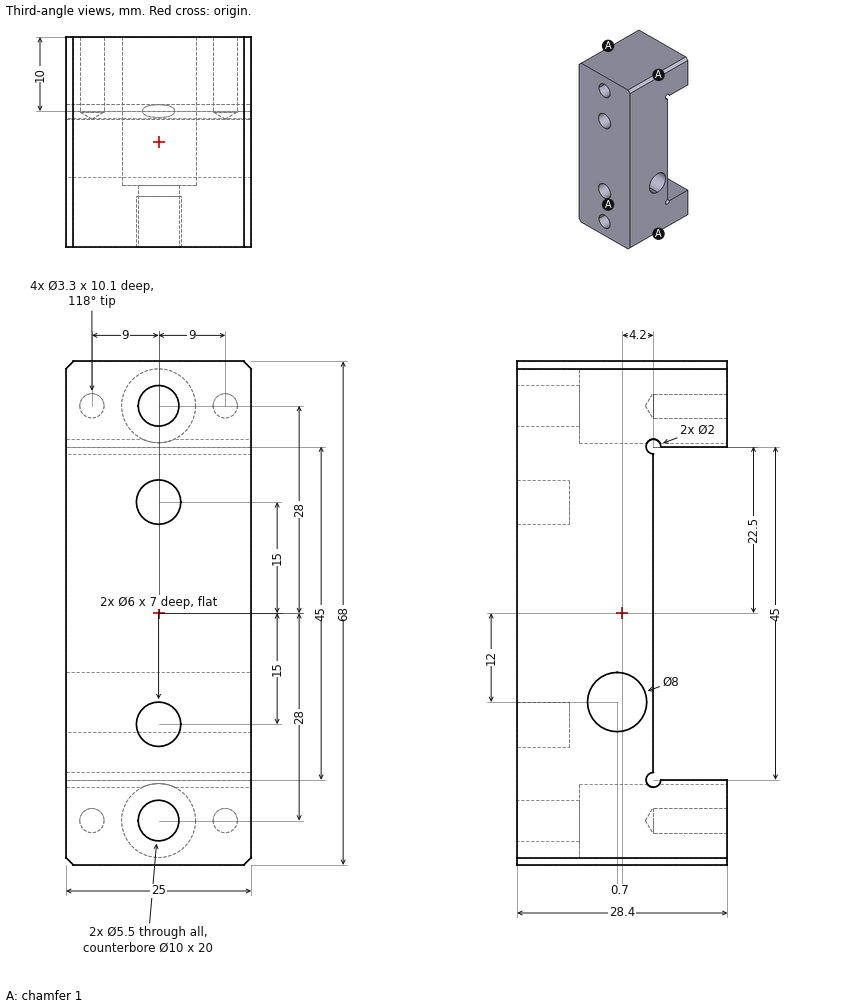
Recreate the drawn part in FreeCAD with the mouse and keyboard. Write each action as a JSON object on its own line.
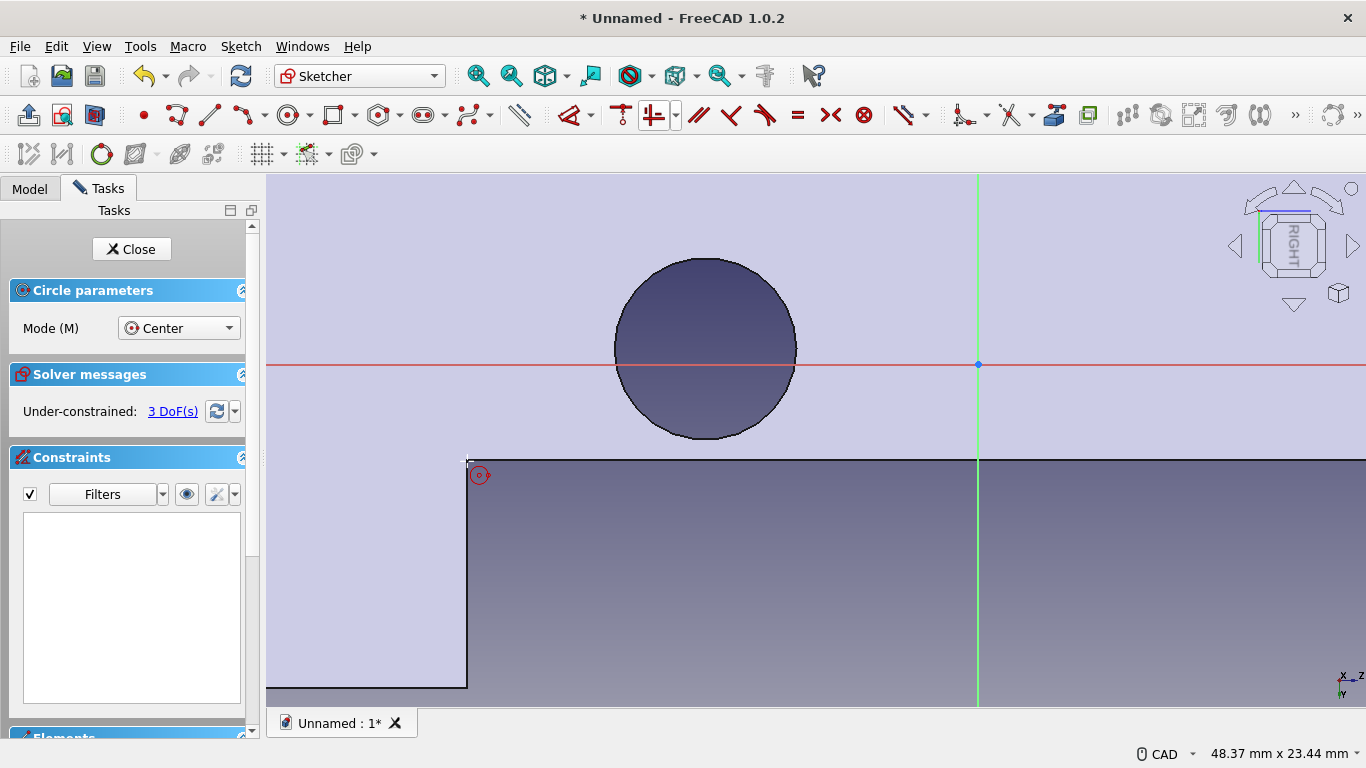
{"action": "left_click", "coordinate": [467, 460]}
{"action": "left_click", "coordinate": [483, 444]}
{"action": "key", "text": "Escape"}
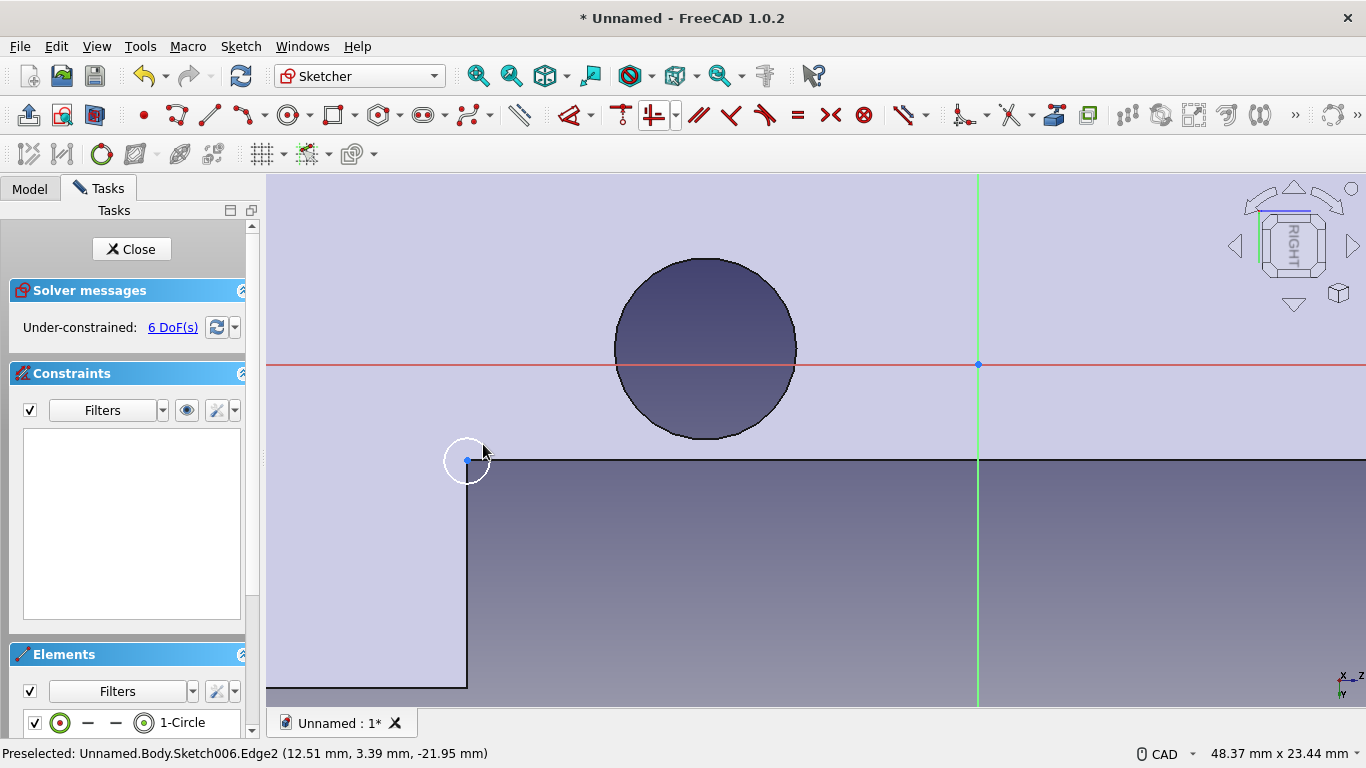
{"action": "scroll", "coordinate": [467, 461], "scroll_direction": "down", "scroll_amount": 3}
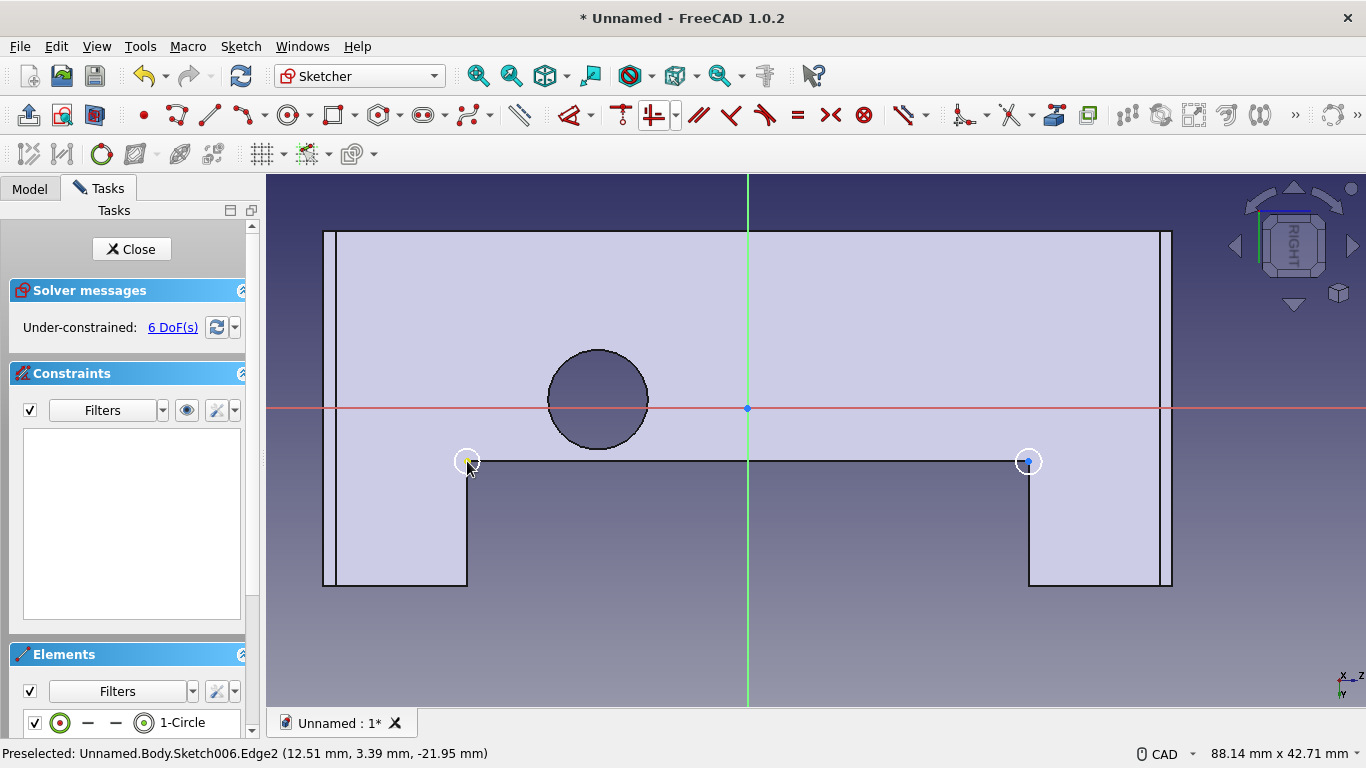
{"action": "left_click", "coordinate": [1038, 453]}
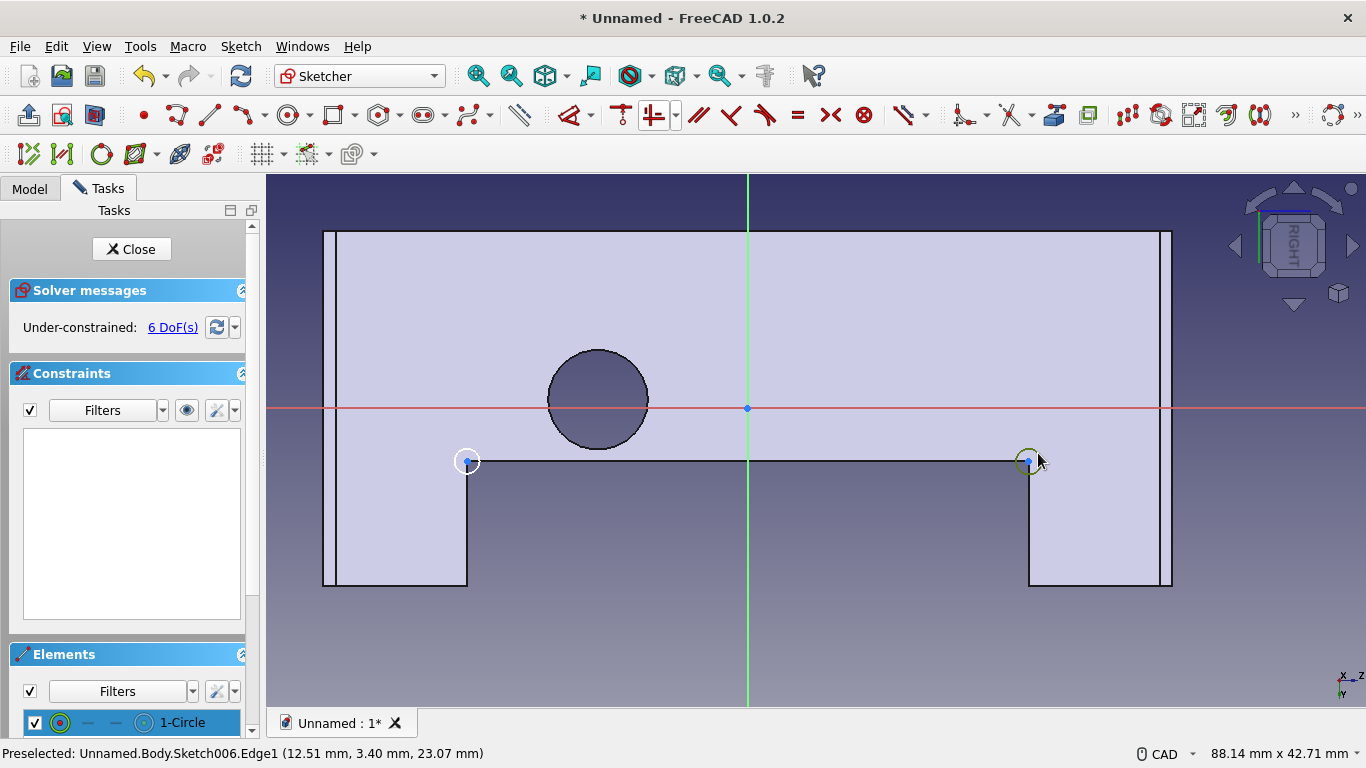
{"action": "left_click", "coordinate": [476, 452]}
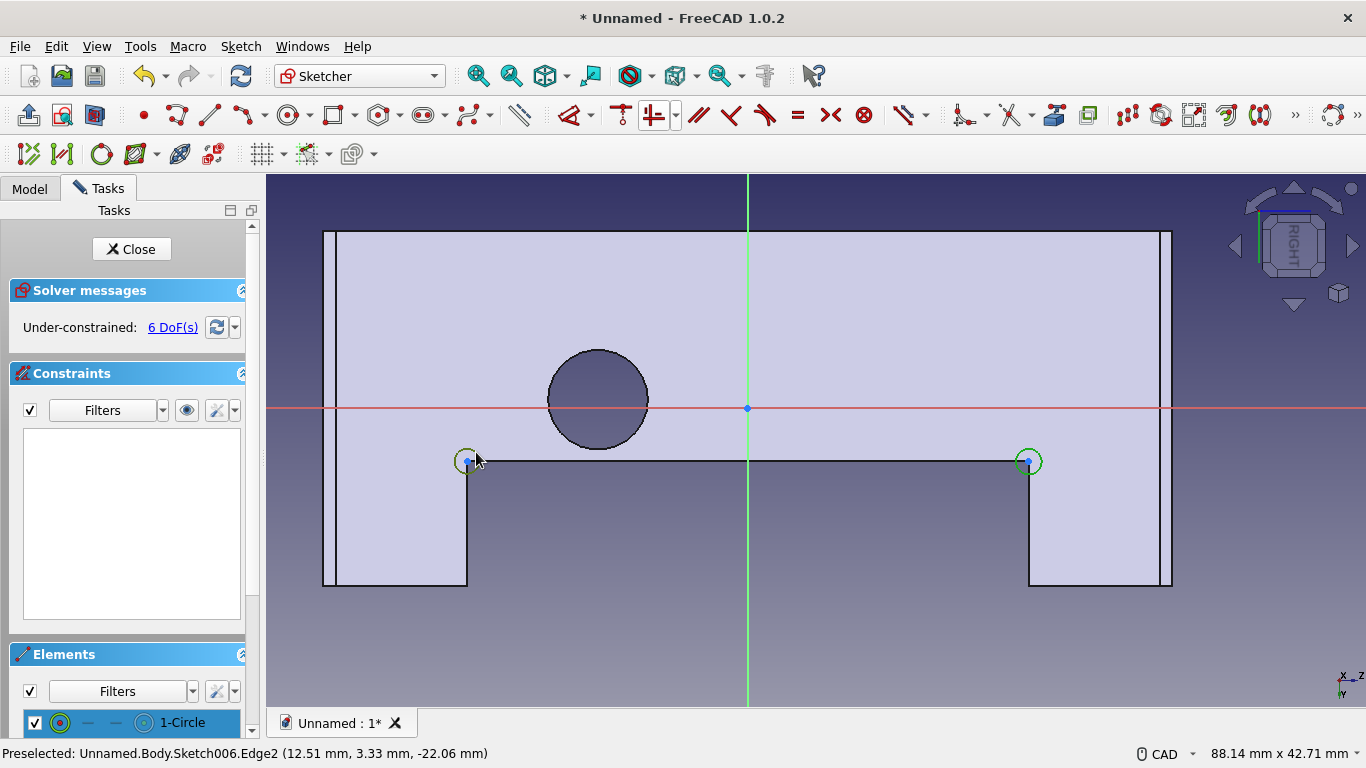
{"action": "key", "text": "e"}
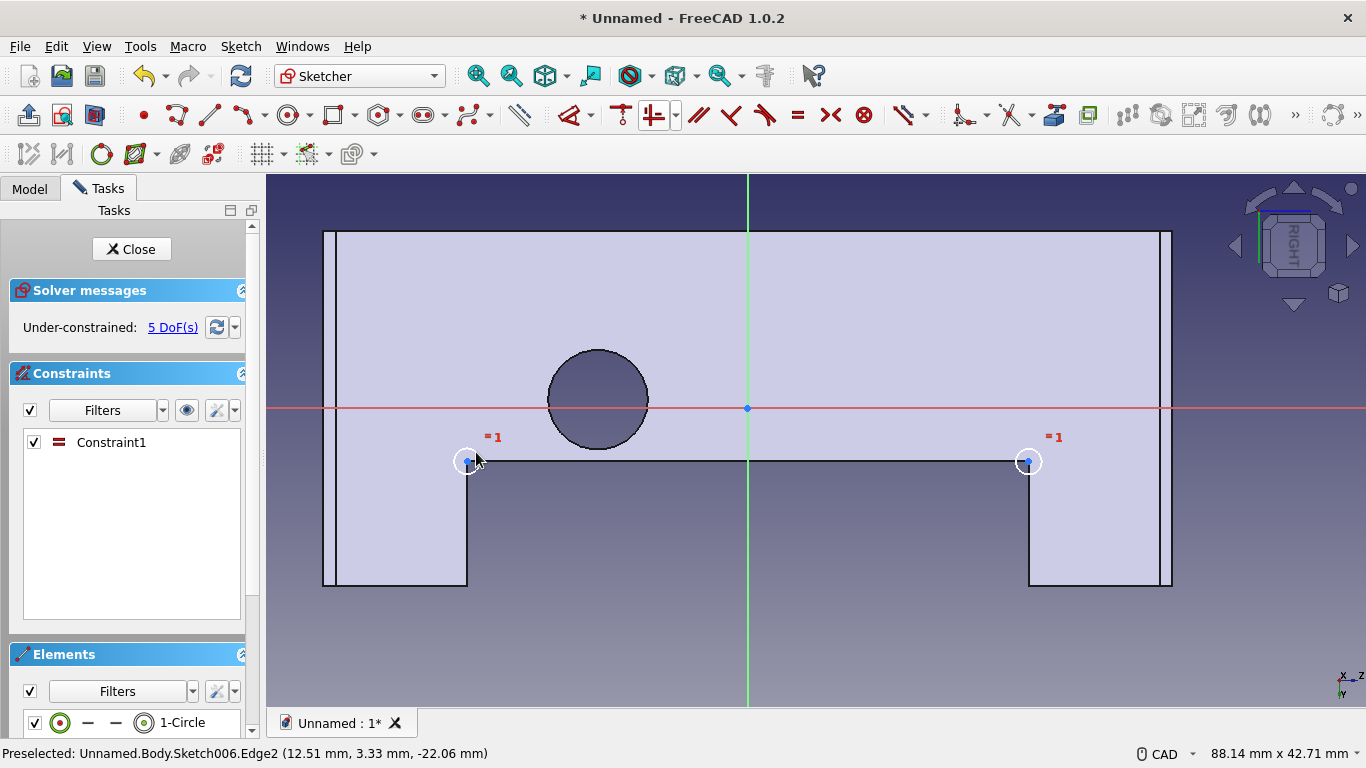
{"action": "left_click", "coordinate": [1029, 462]}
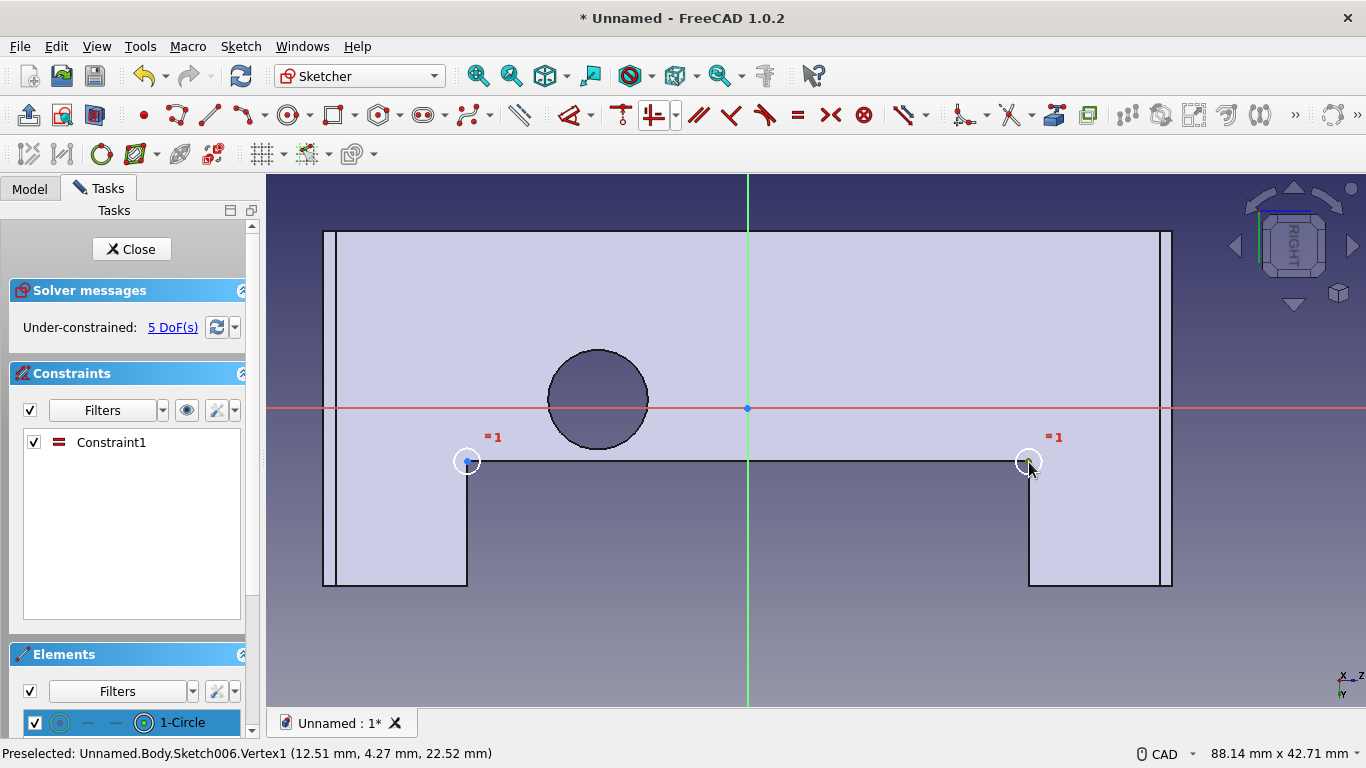
{"action": "left_click", "coordinate": [467, 461]}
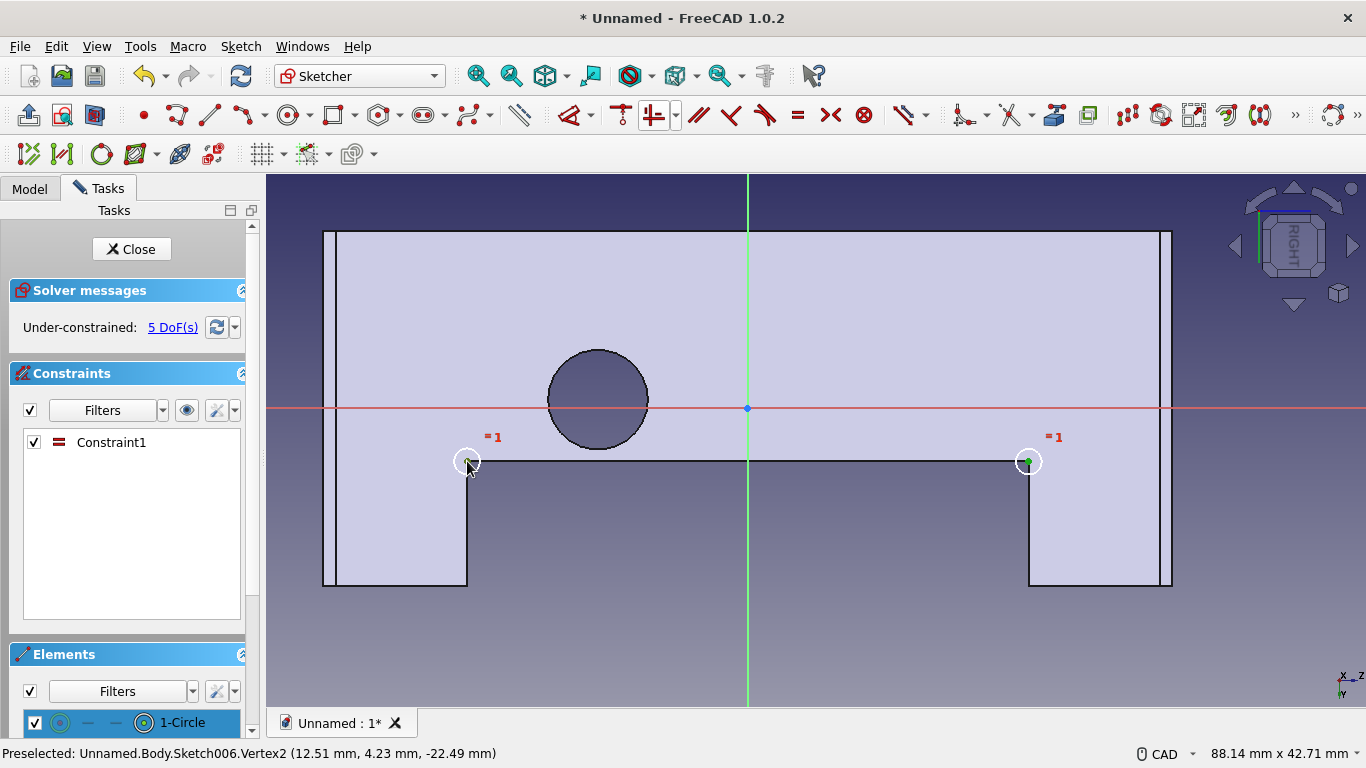
{"action": "key", "text": "h"}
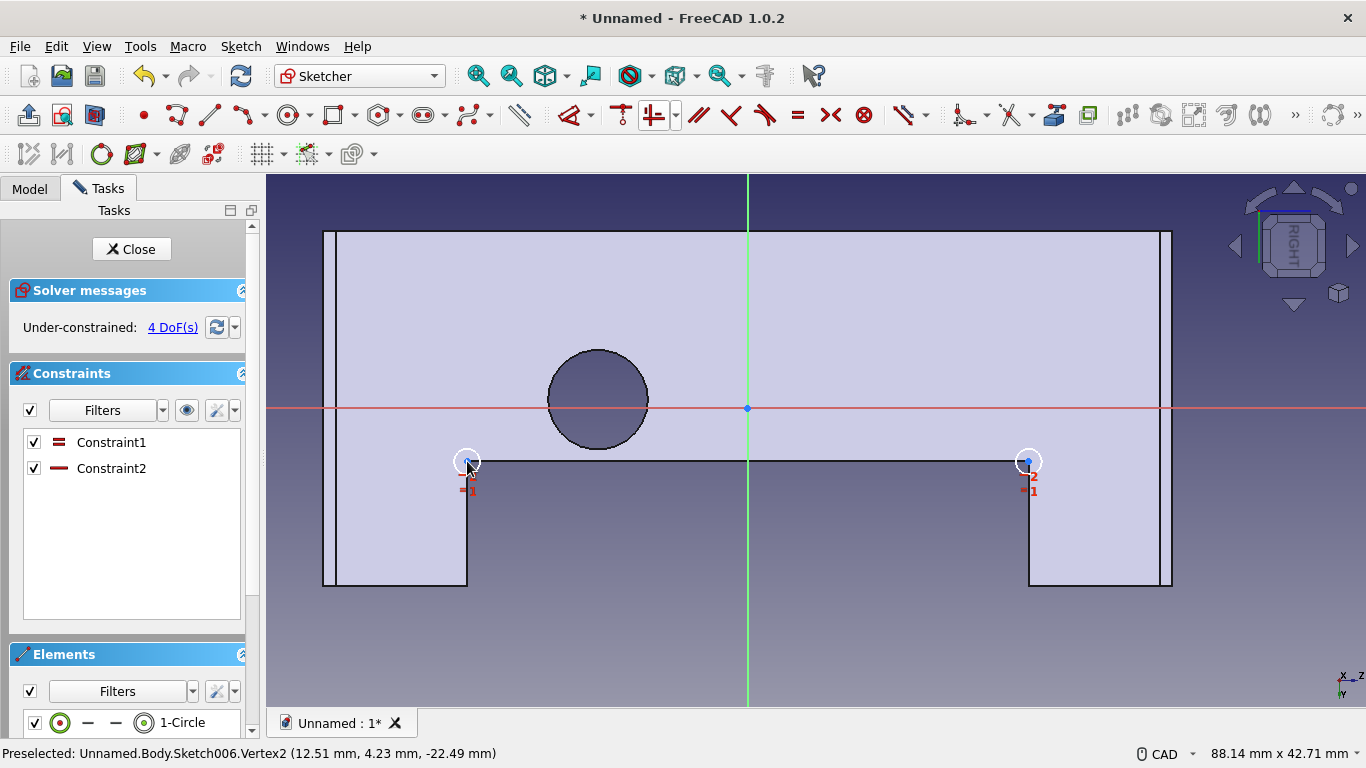
{"action": "left_click", "coordinate": [568, 116]}